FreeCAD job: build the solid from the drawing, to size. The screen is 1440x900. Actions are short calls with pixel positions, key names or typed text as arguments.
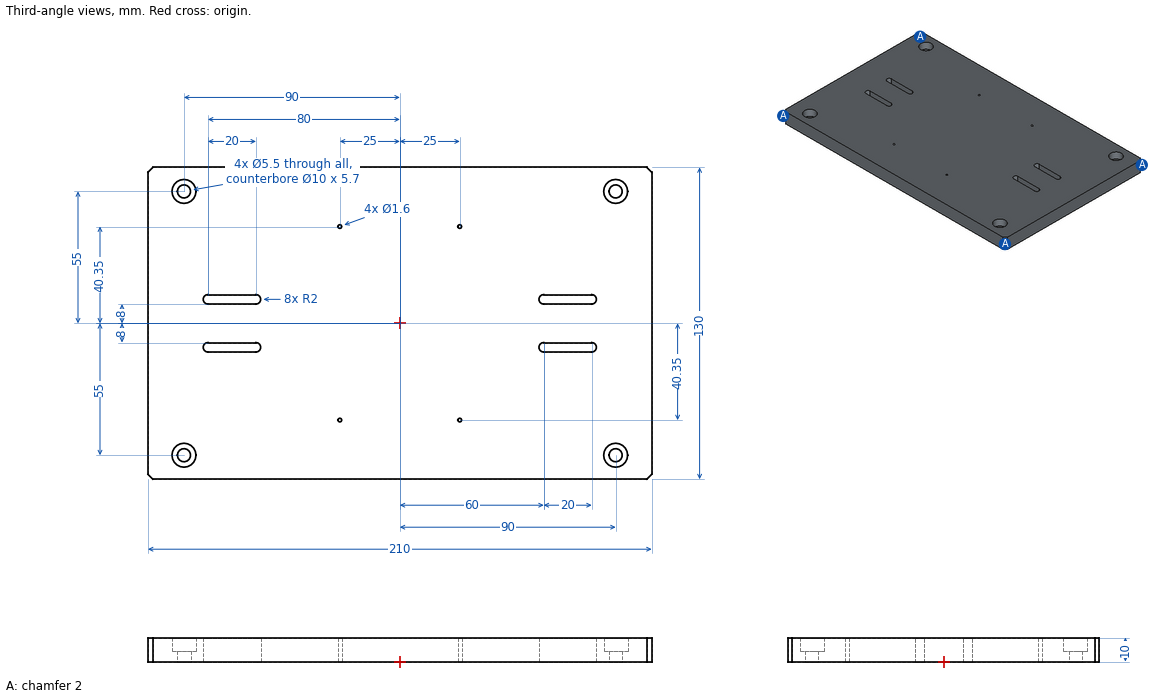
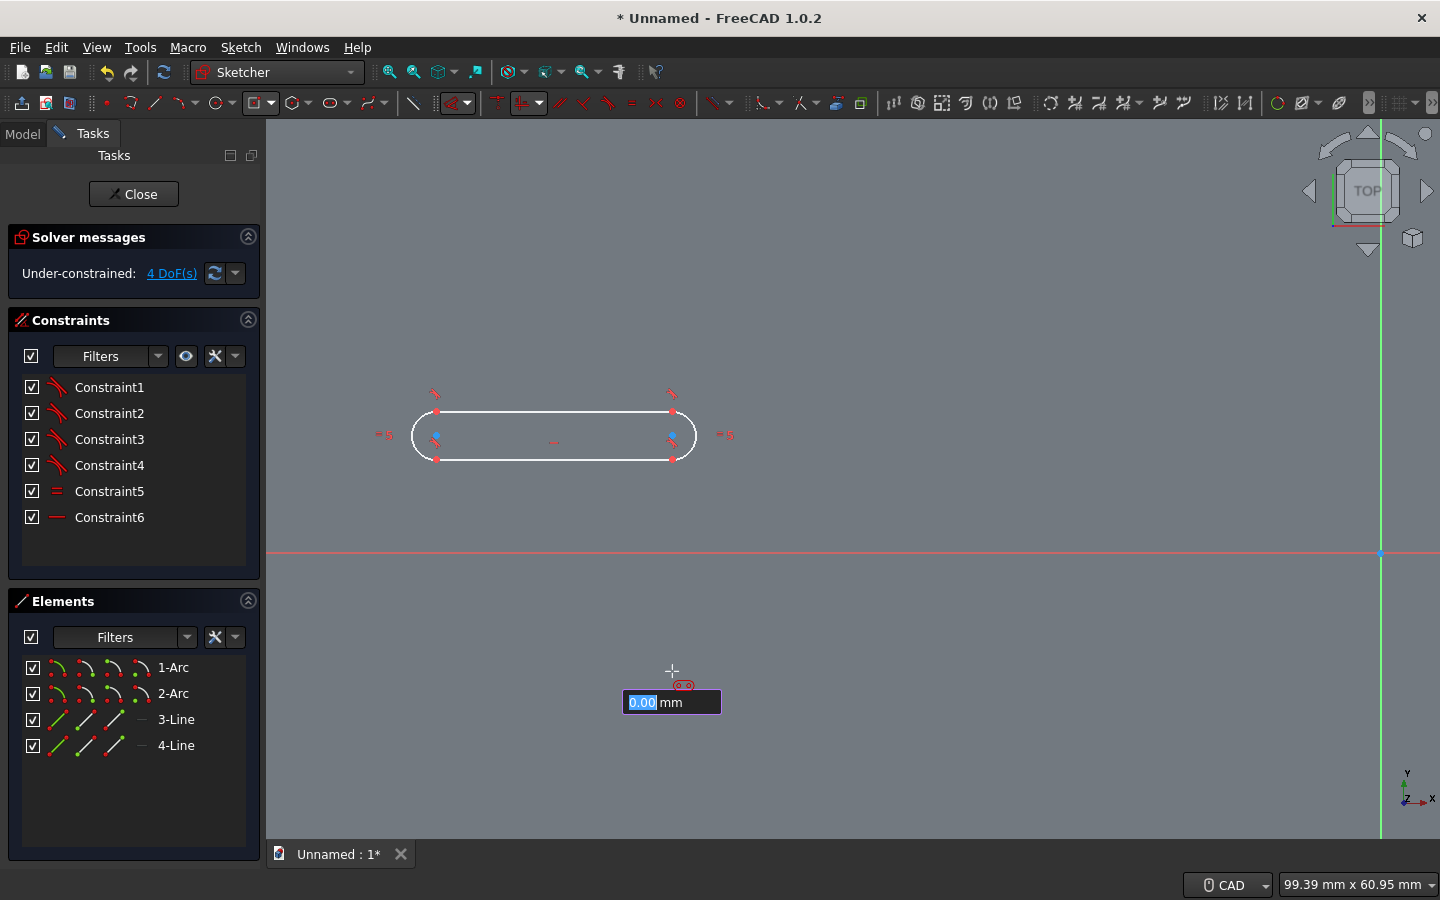
click(554, 648)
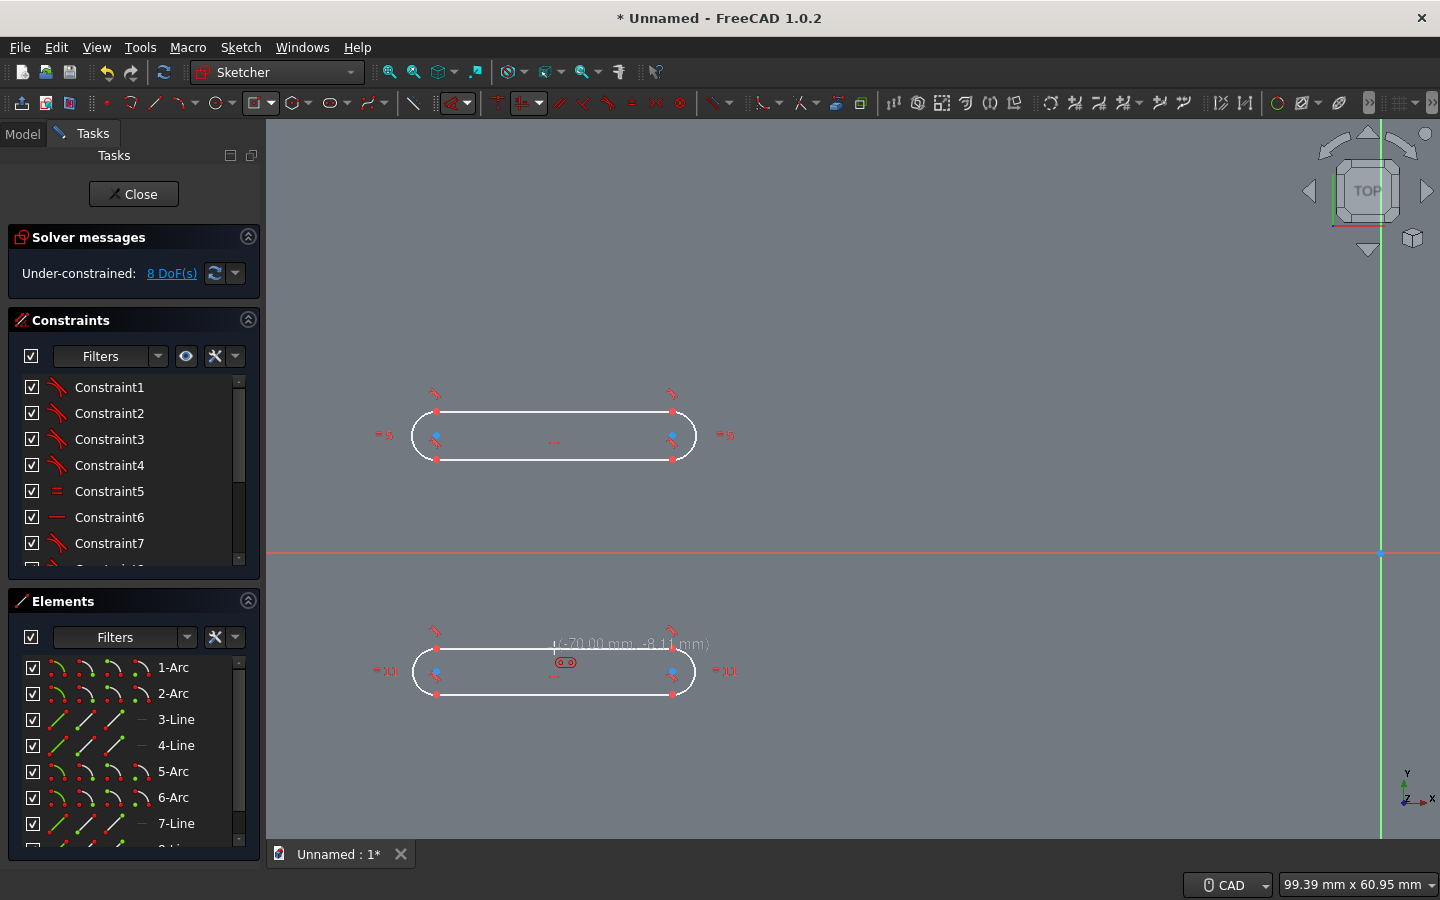
scroll(437, 436, down, 5)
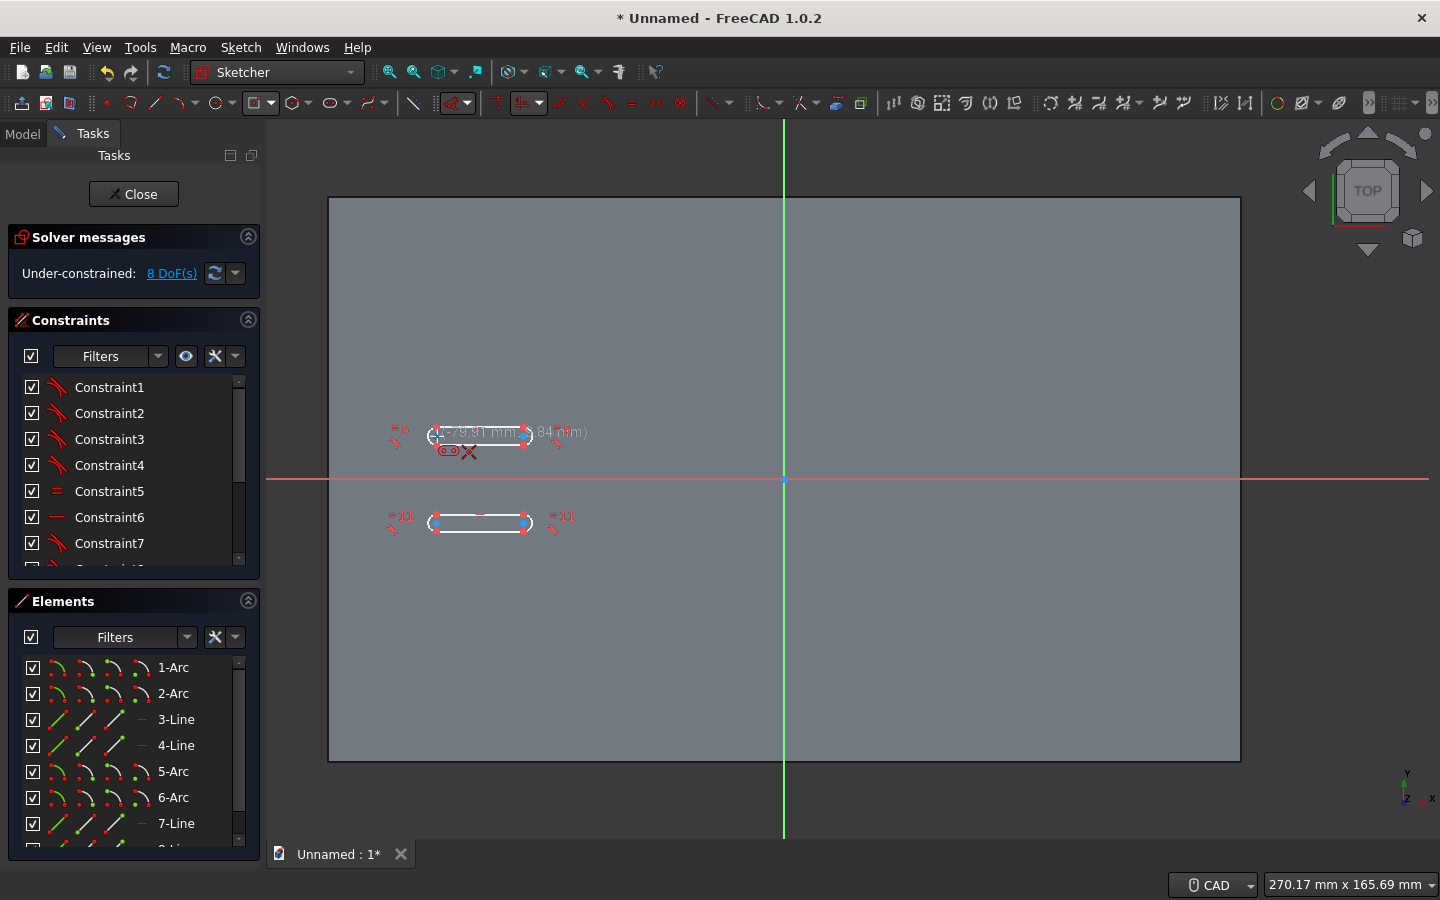
scroll(1045, 523, up, 5)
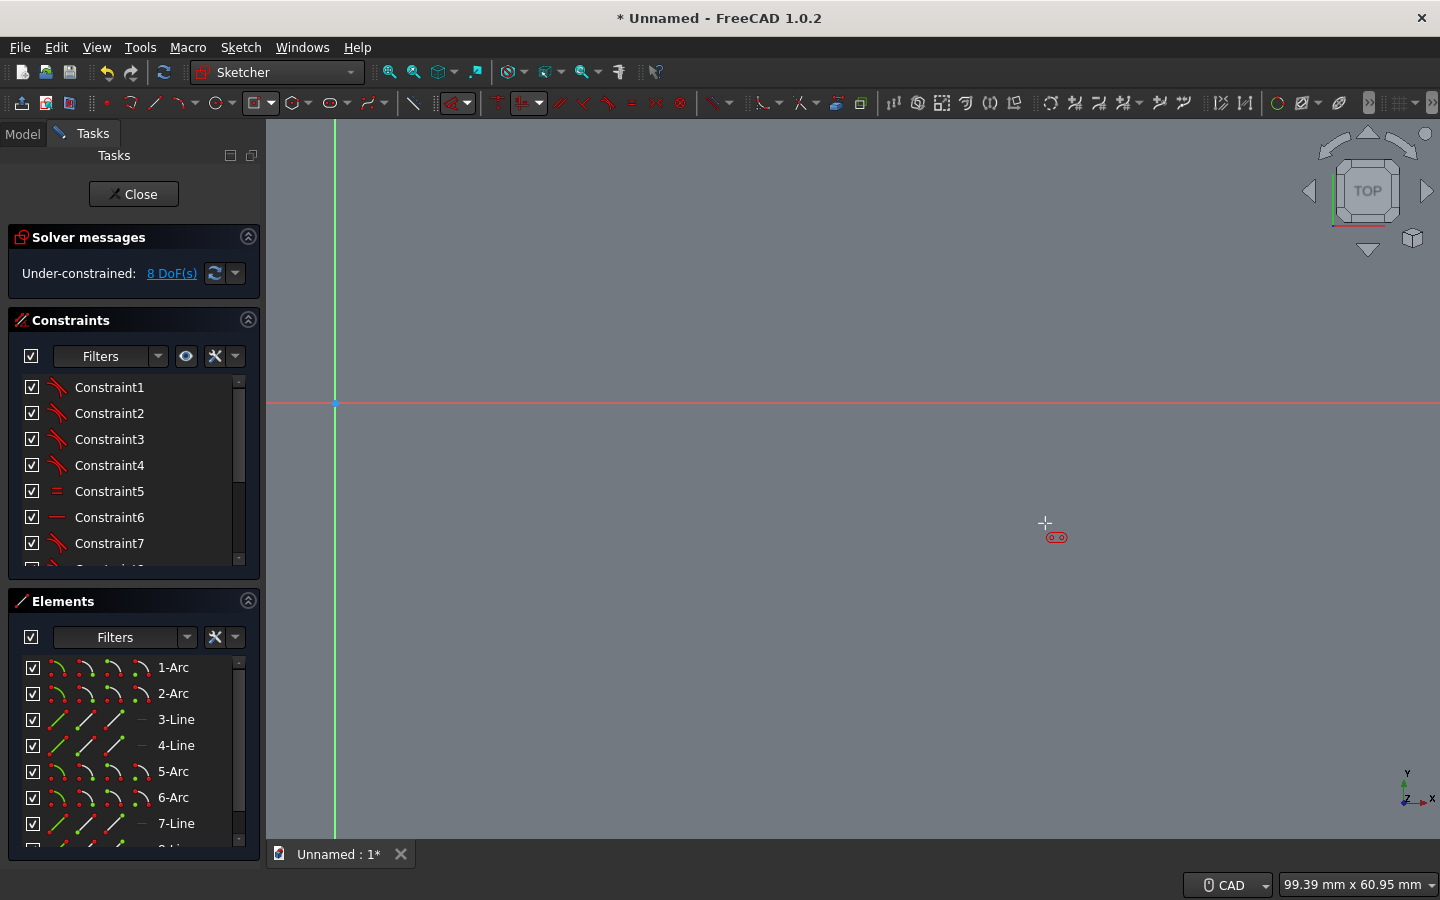
click(1044, 522)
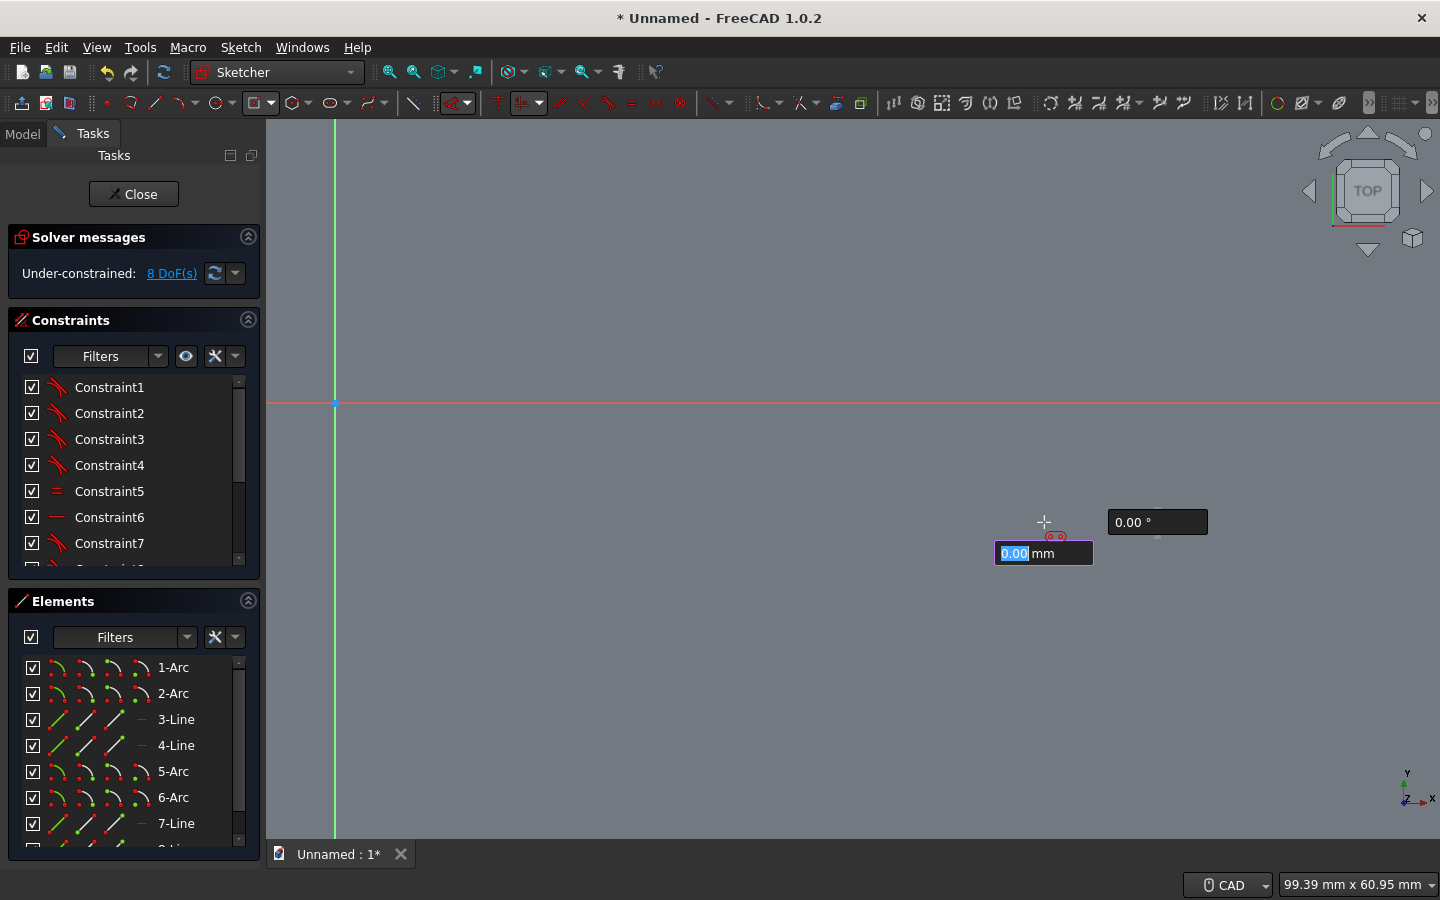
scroll(1046, 523, down, 5)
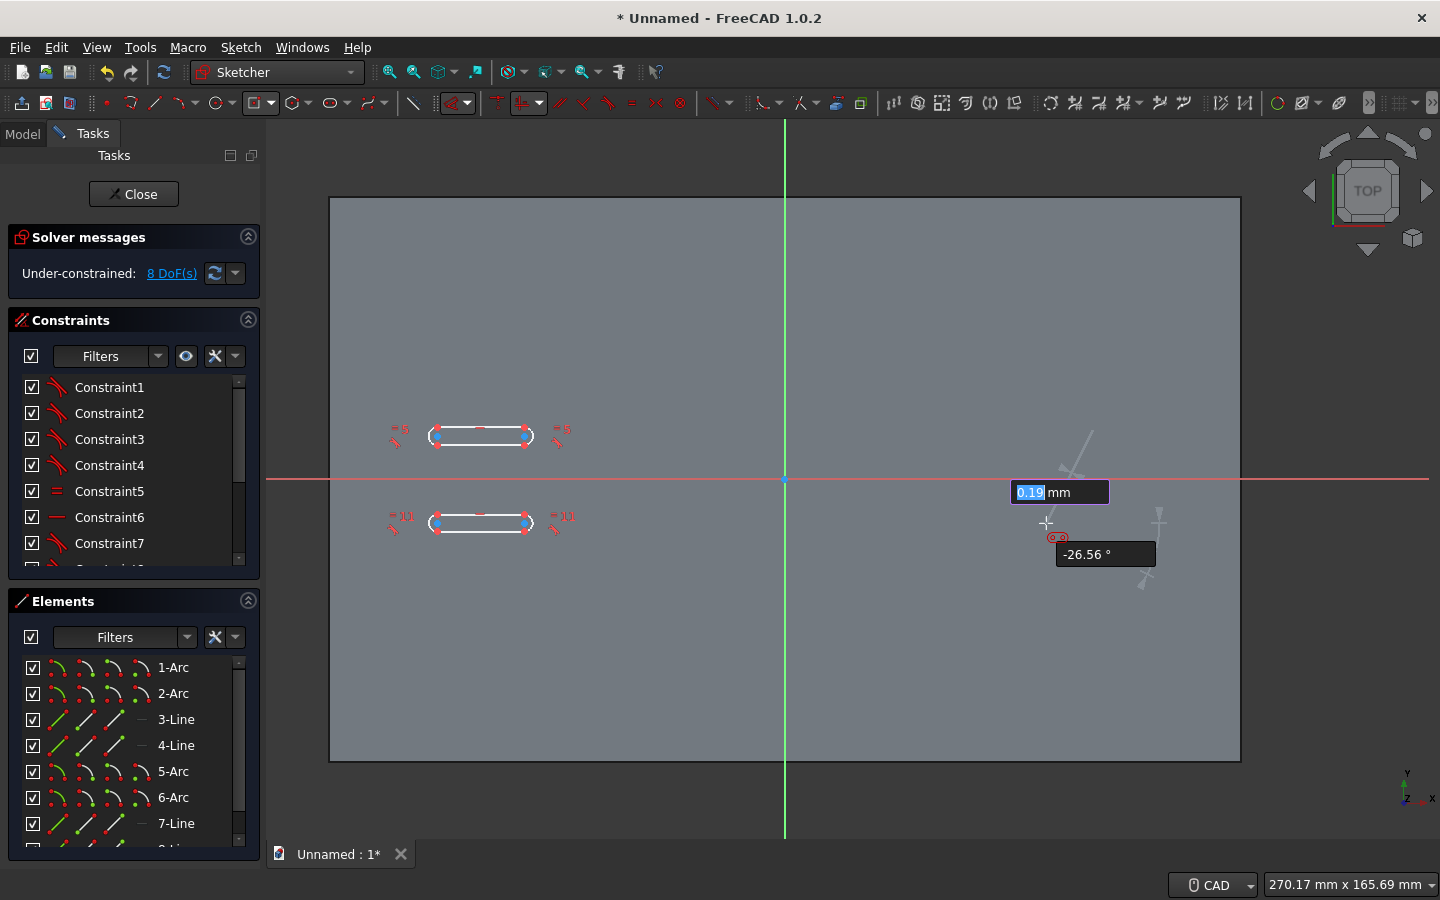
click(1133, 523)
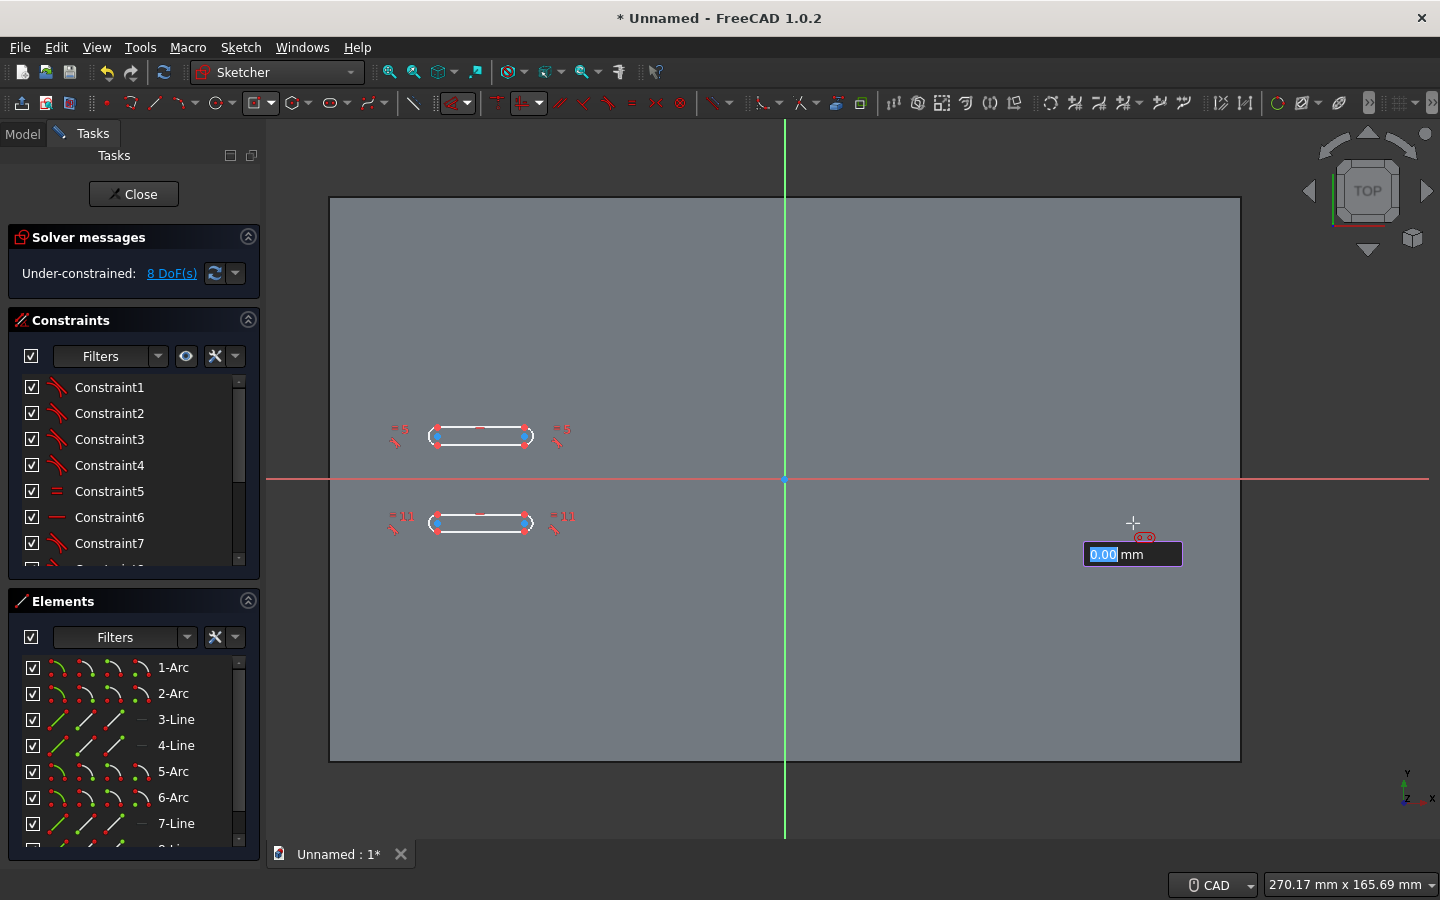
scroll(1089, 514, up, 4)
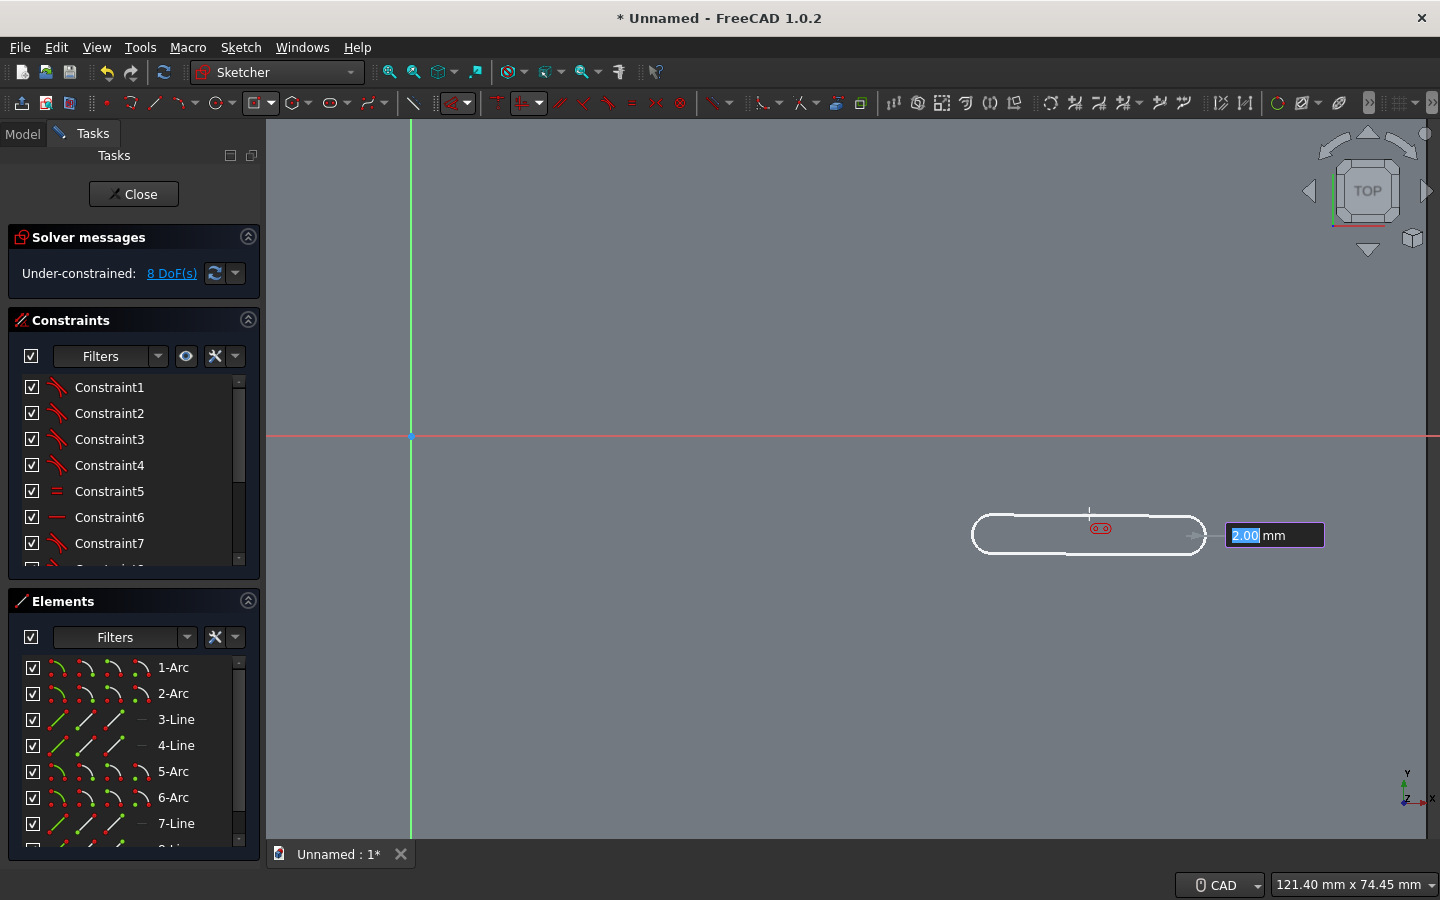
click(1088, 514)